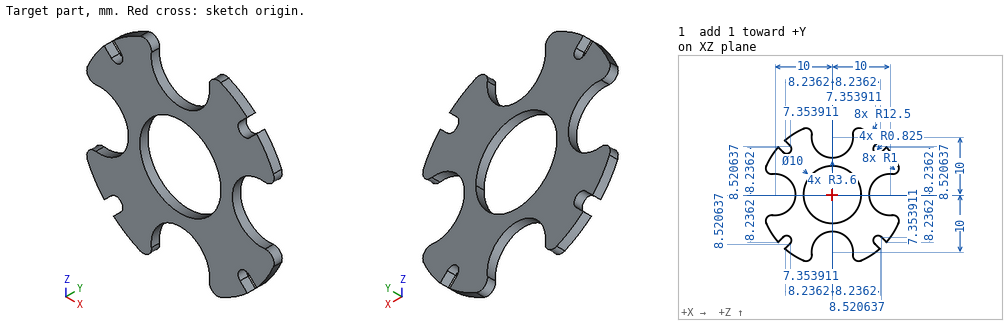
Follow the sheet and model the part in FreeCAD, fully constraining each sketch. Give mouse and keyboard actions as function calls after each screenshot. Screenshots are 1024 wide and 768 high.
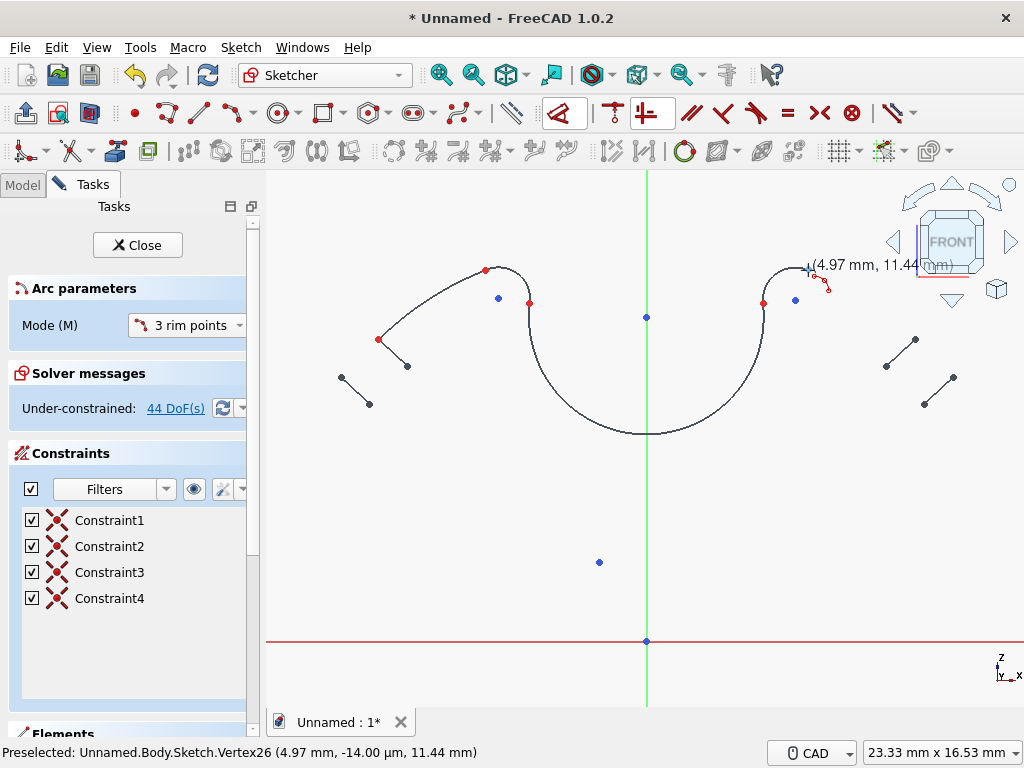
scroll(519, 273, down, 4)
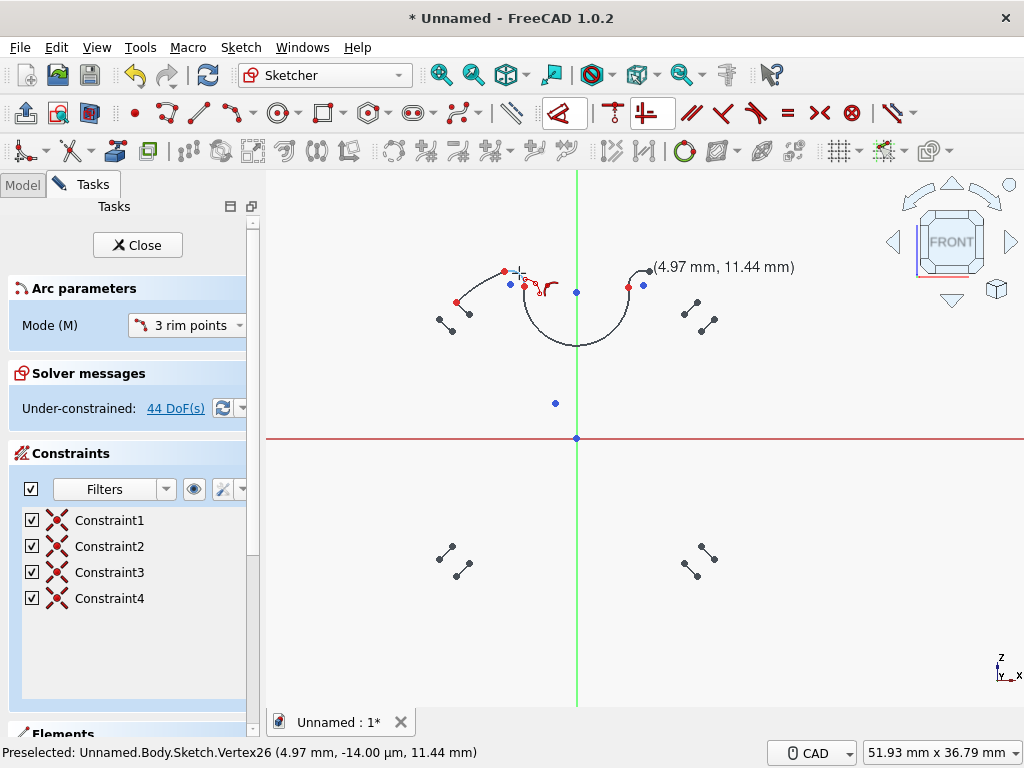
scroll(697, 302, up, 3)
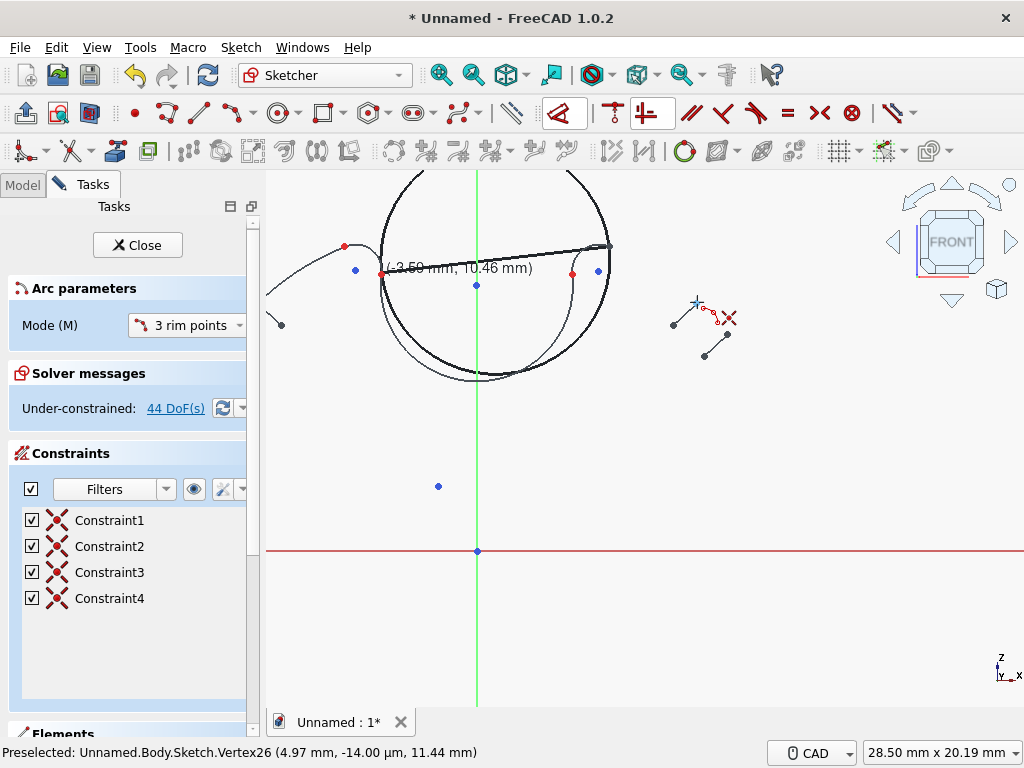
click(697, 304)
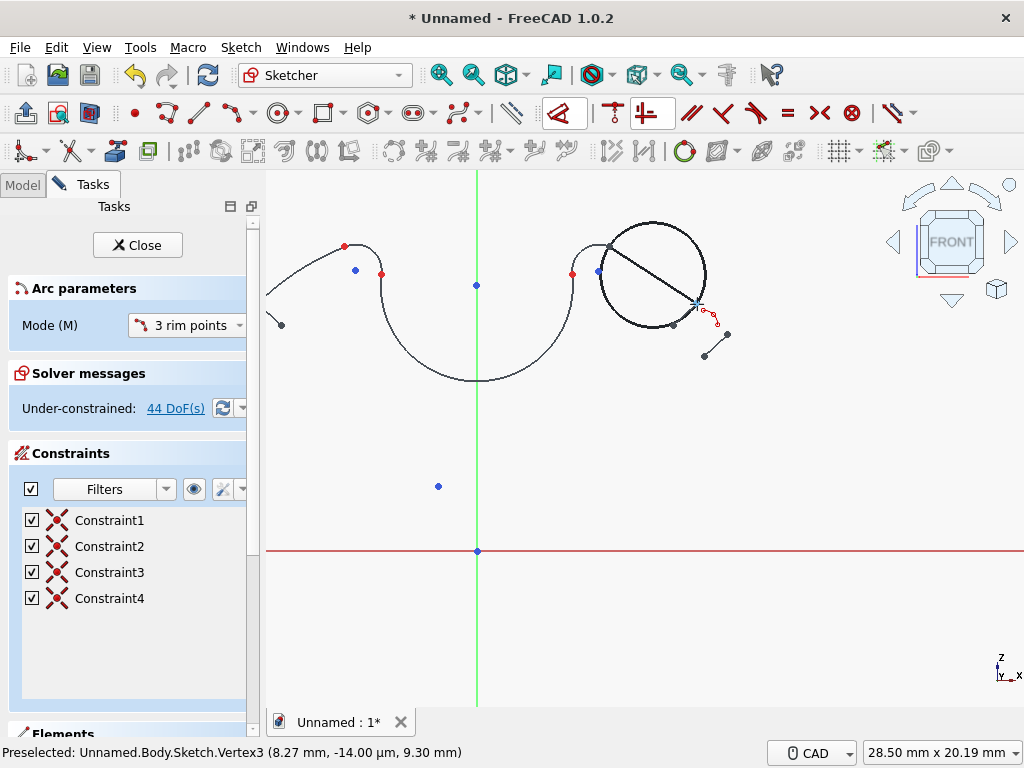
scroll(655, 270, up, 7)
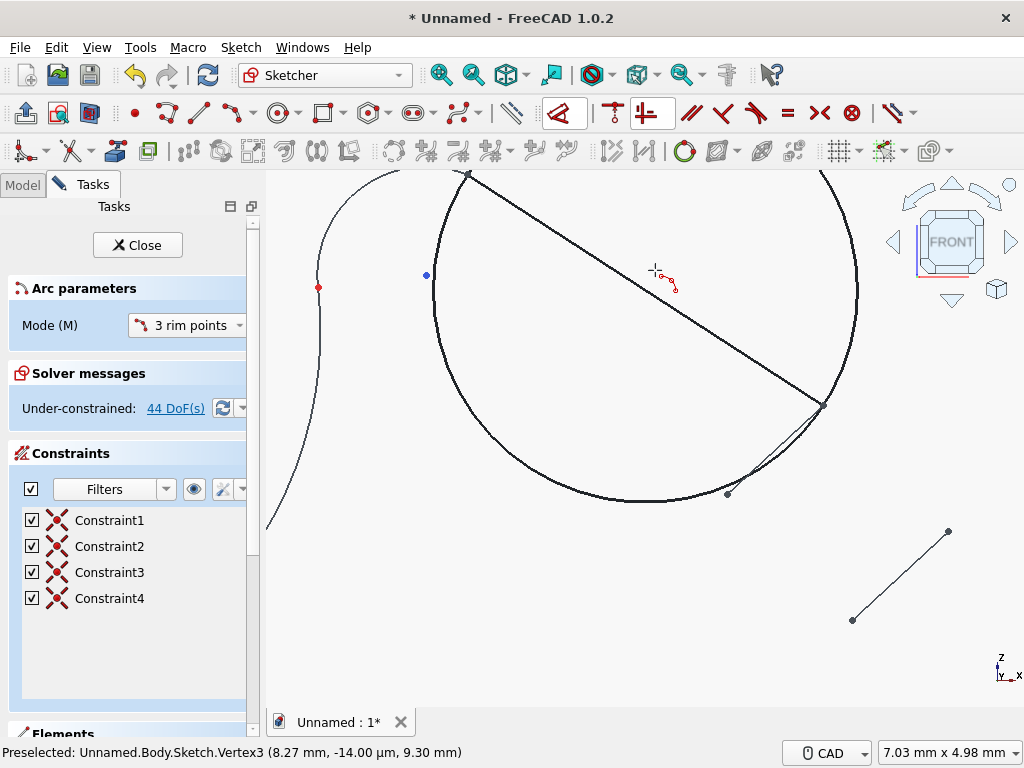
click(652, 269)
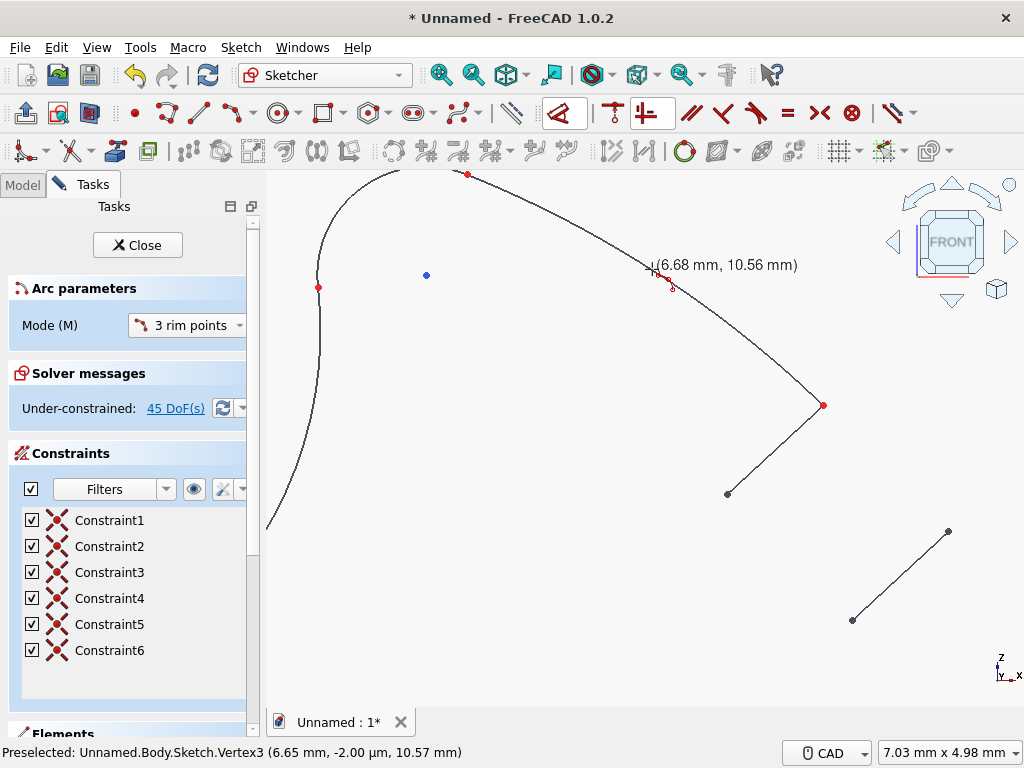
scroll(677, 287, down, 10)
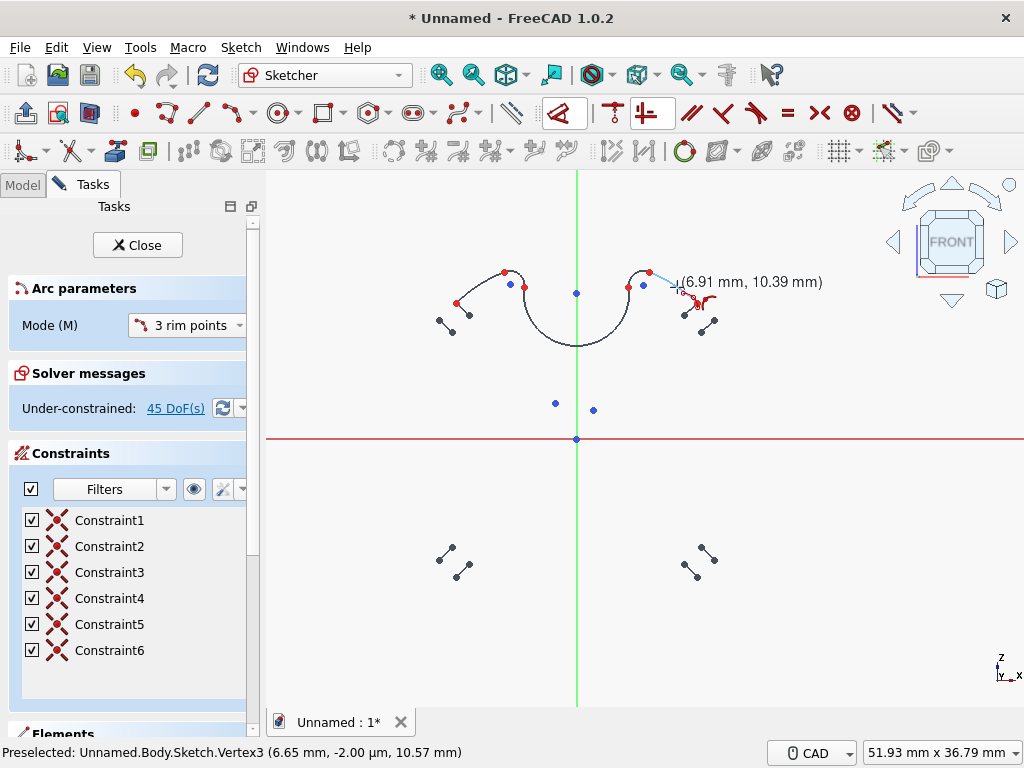
scroll(684, 315, up, 3)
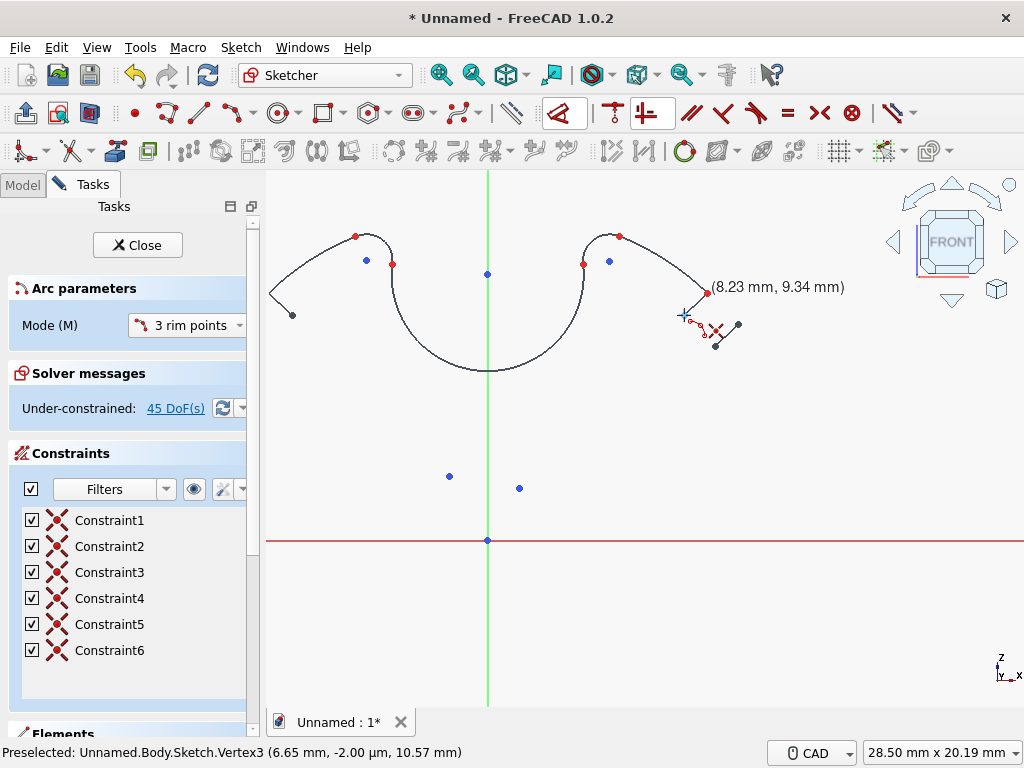
click(684, 315)
click(715, 346)
click(683, 345)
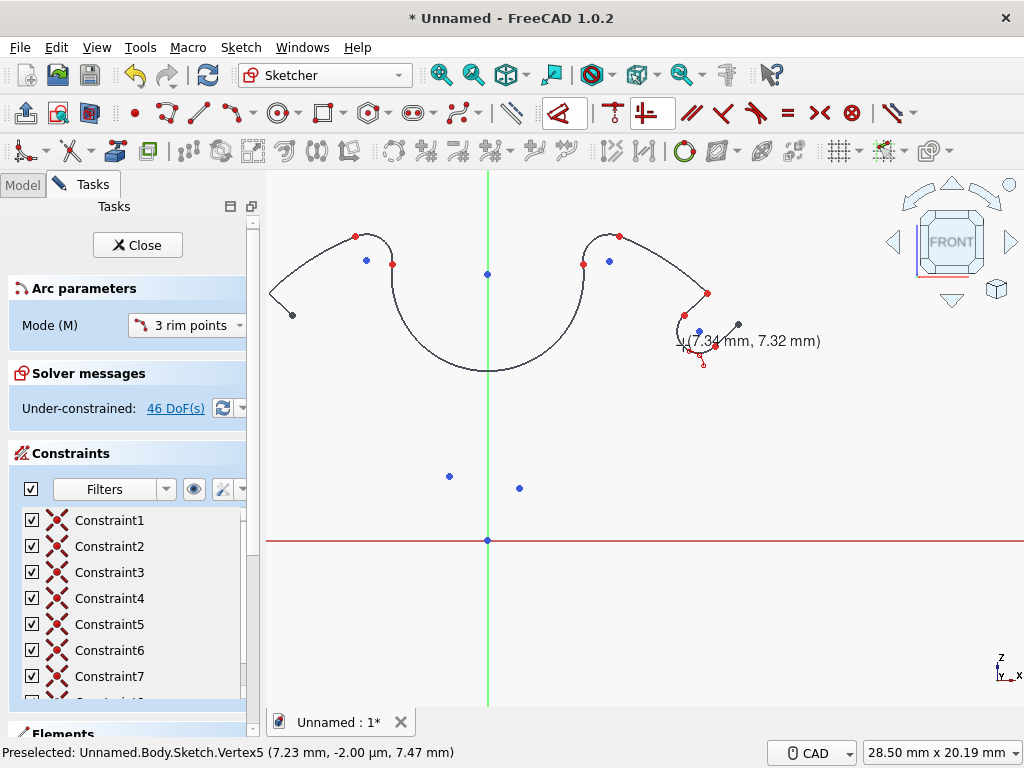
click(739, 324)
click(793, 409)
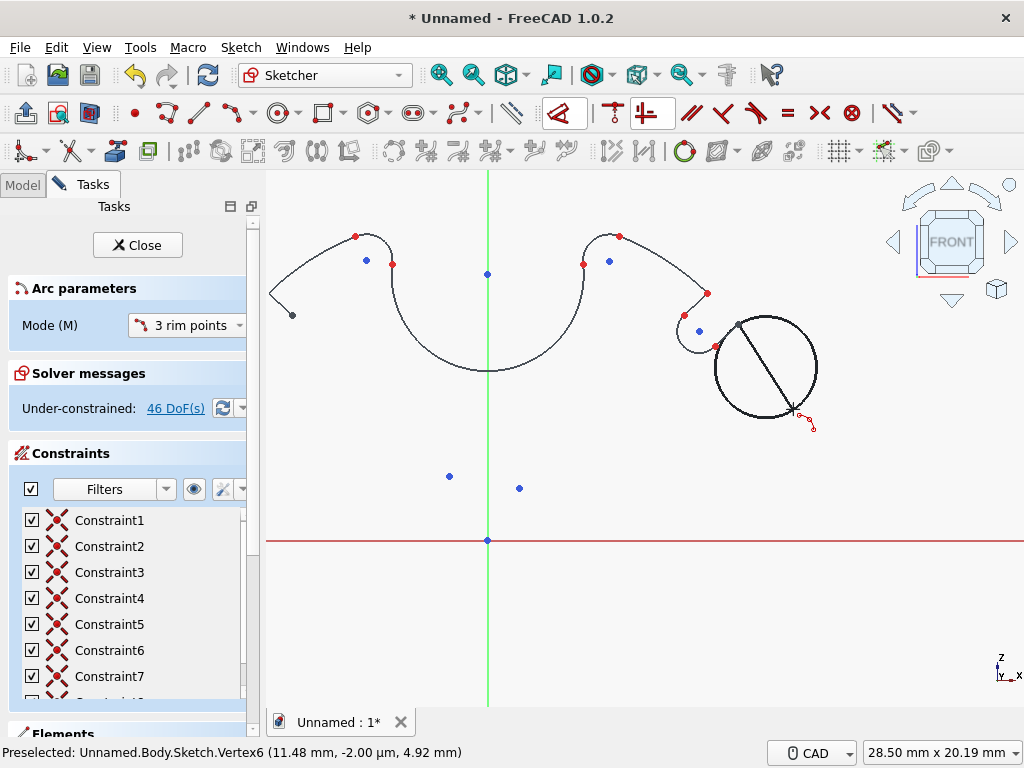
scroll(769, 363, up, 7)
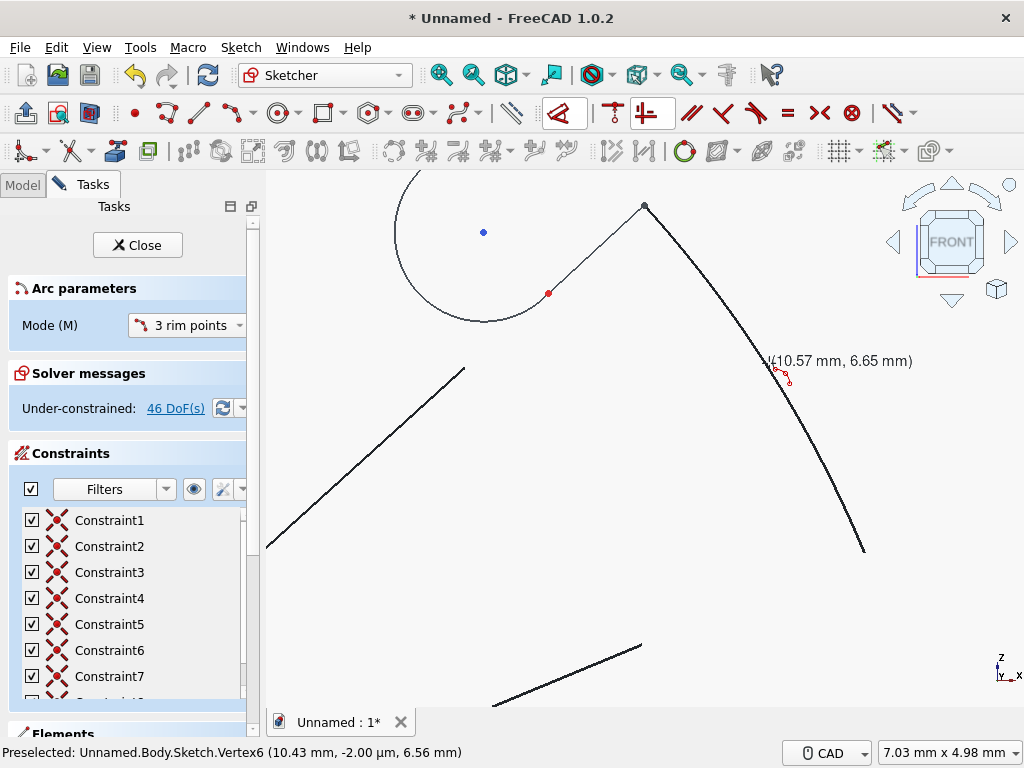
click(766, 362)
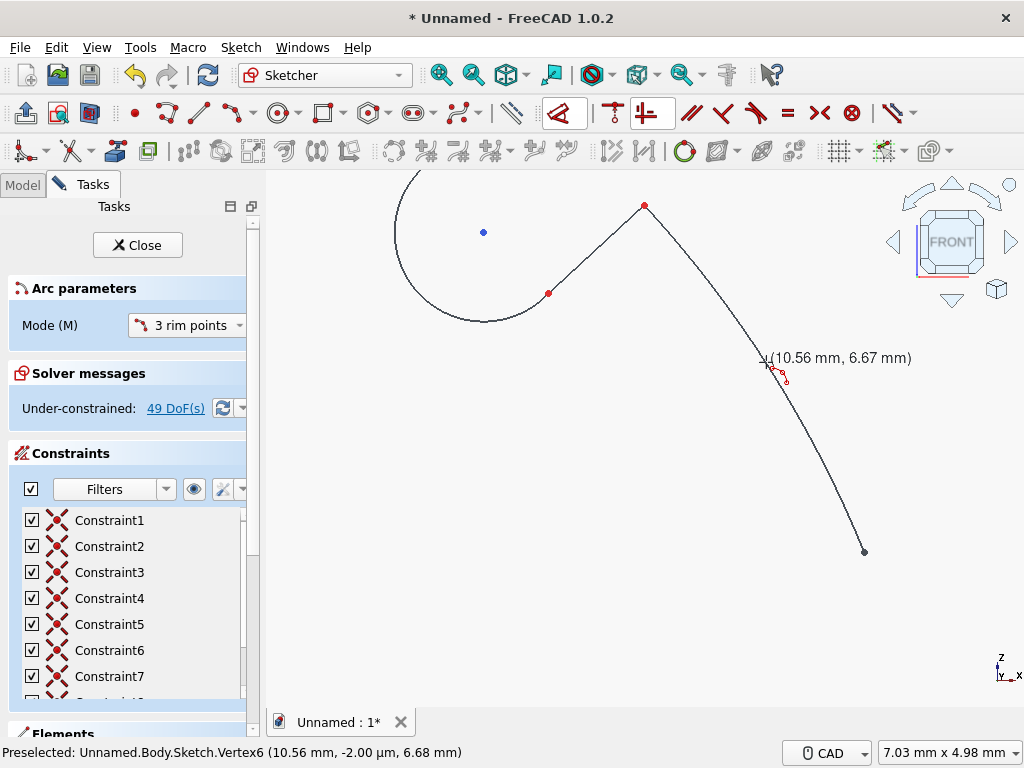
scroll(725, 338, down, 10)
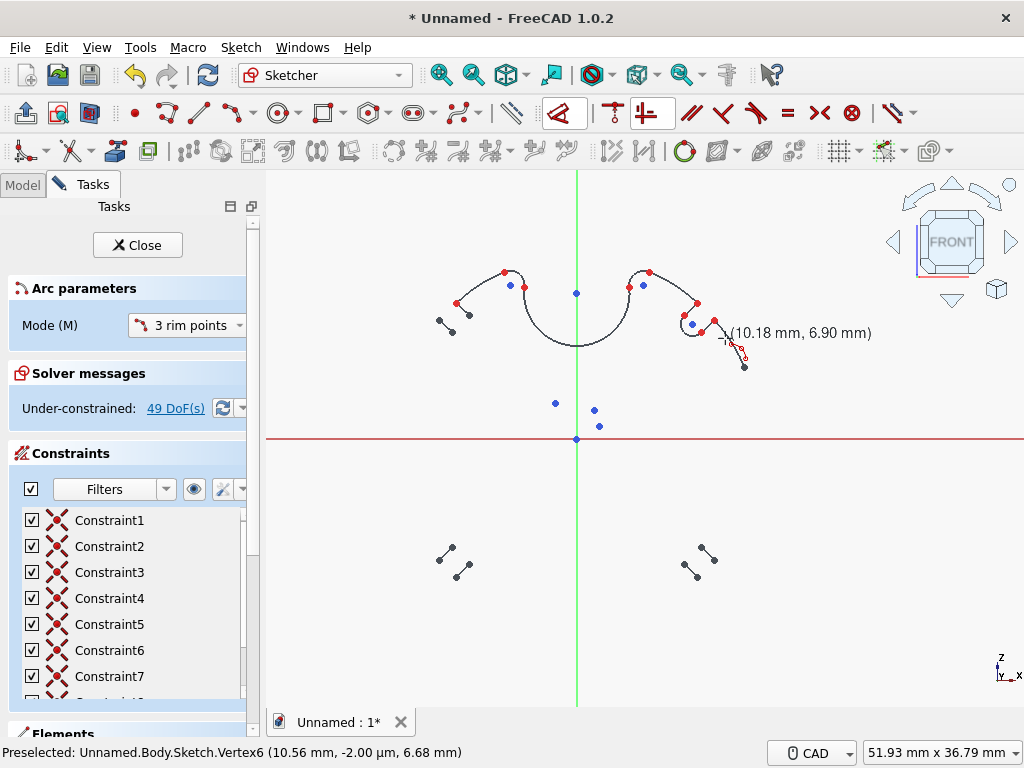
click(744, 367)
click(729, 387)